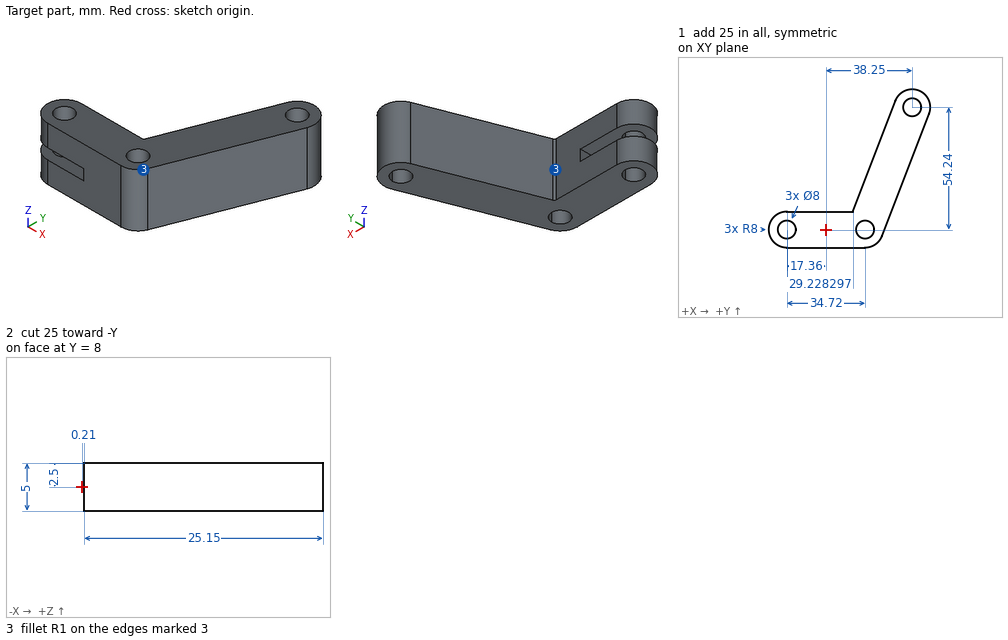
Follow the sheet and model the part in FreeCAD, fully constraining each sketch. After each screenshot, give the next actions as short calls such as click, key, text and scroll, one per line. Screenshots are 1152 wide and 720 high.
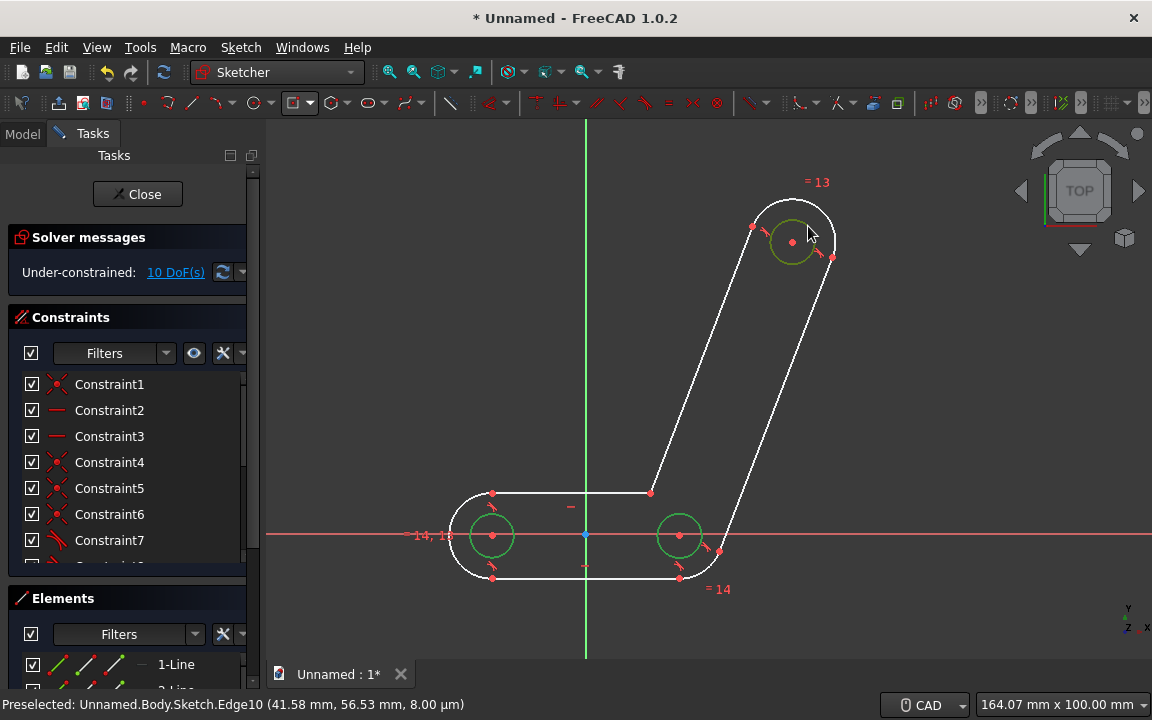
click(670, 104)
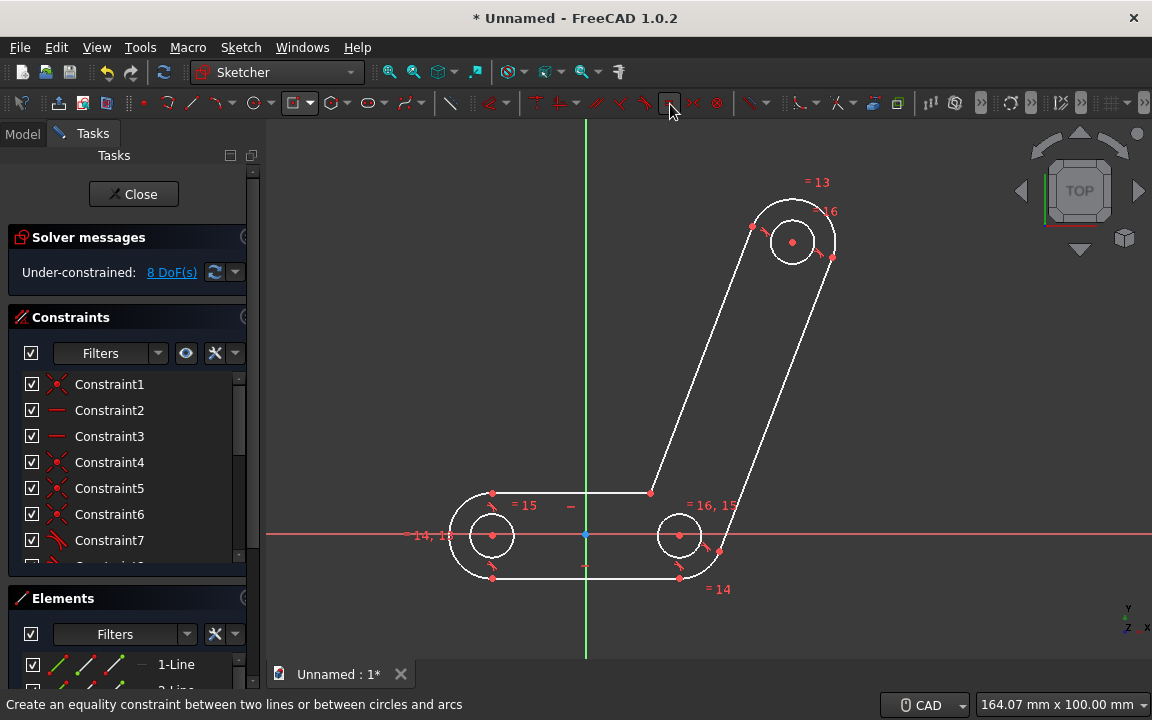
click(492, 536)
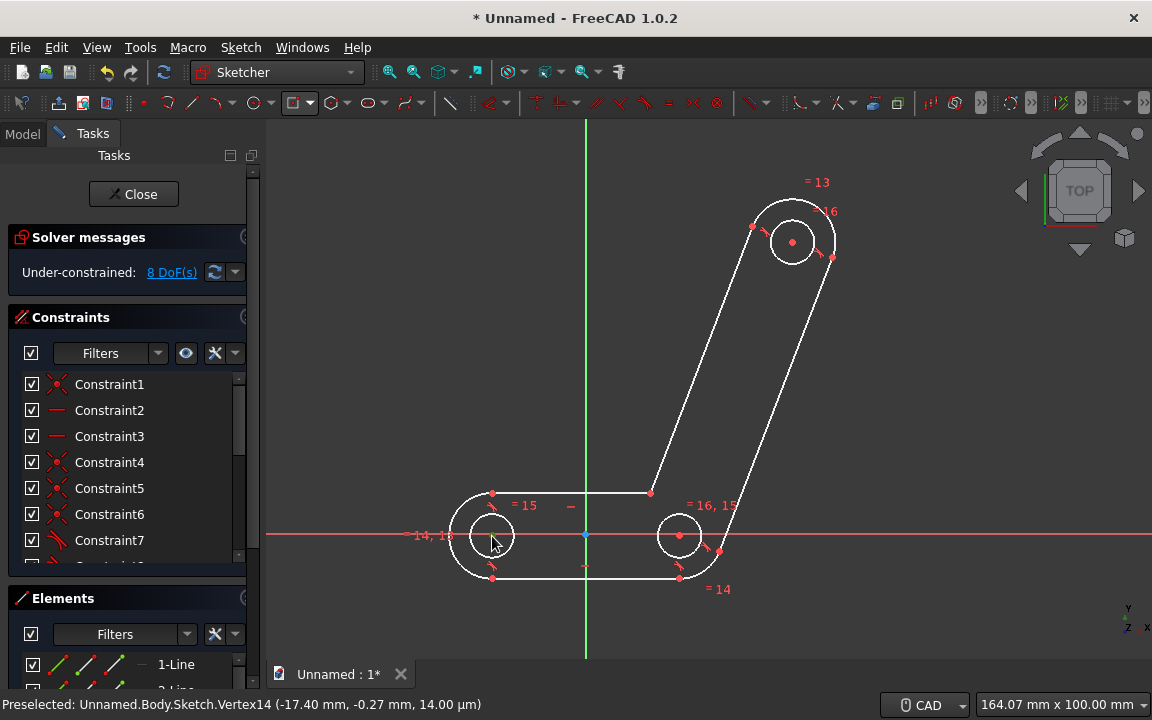
click(344, 534)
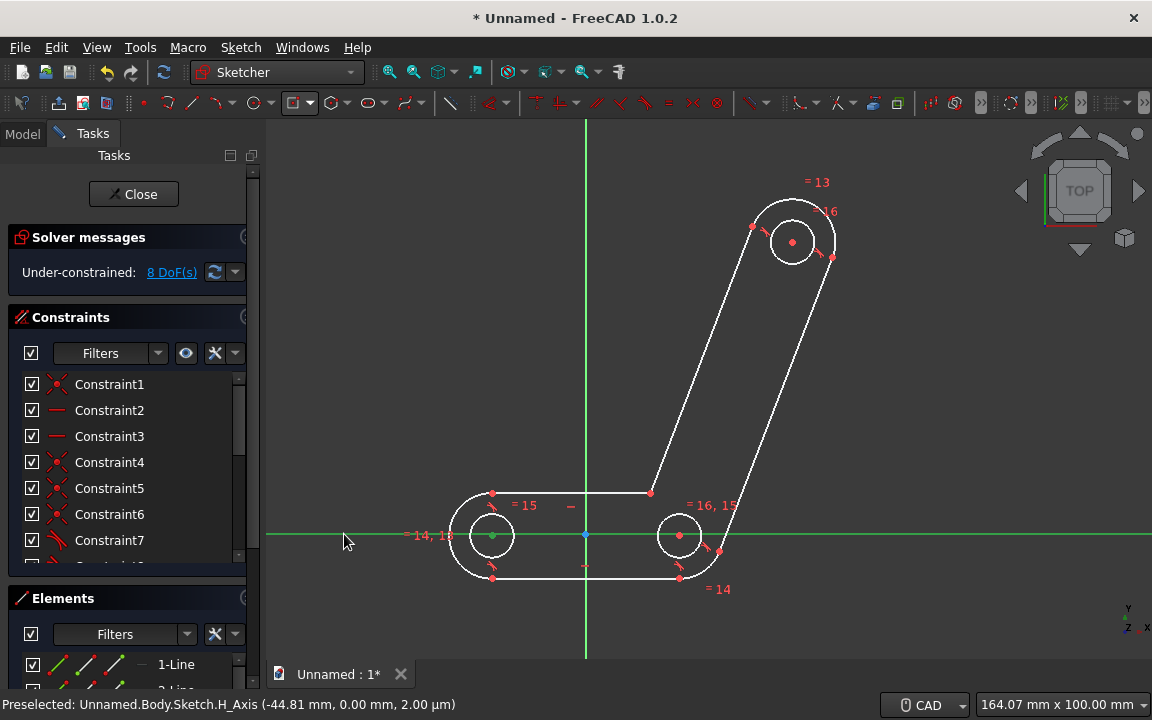
click(536, 104)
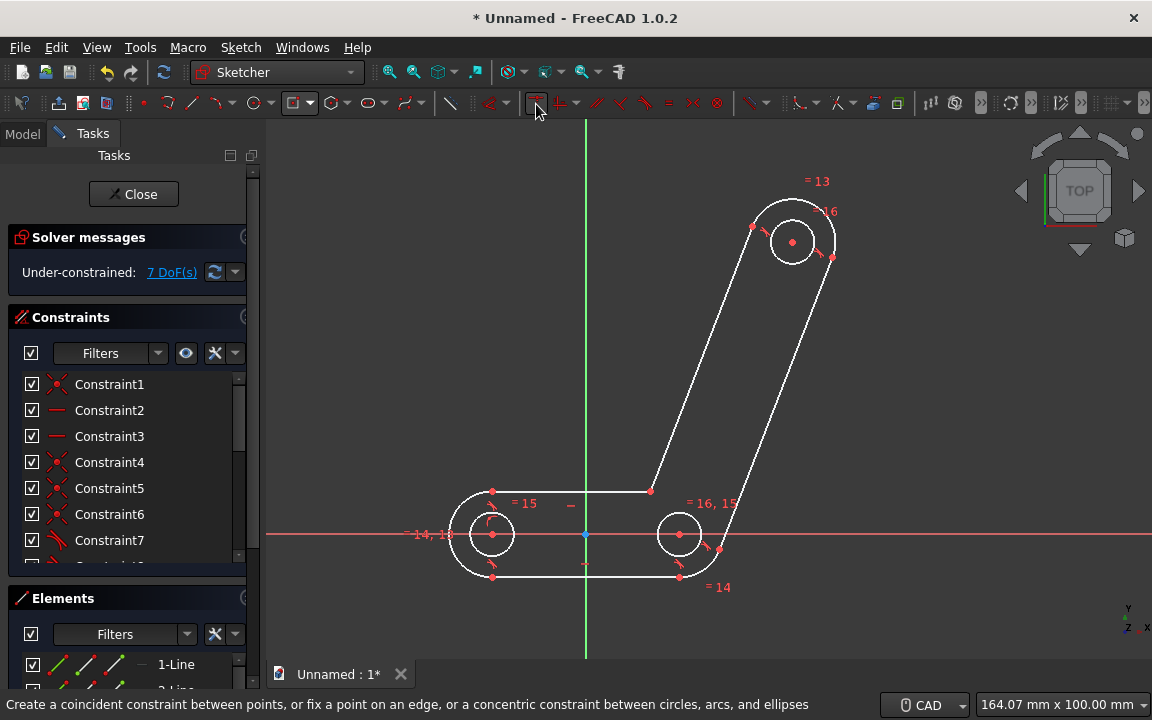
click(829, 219)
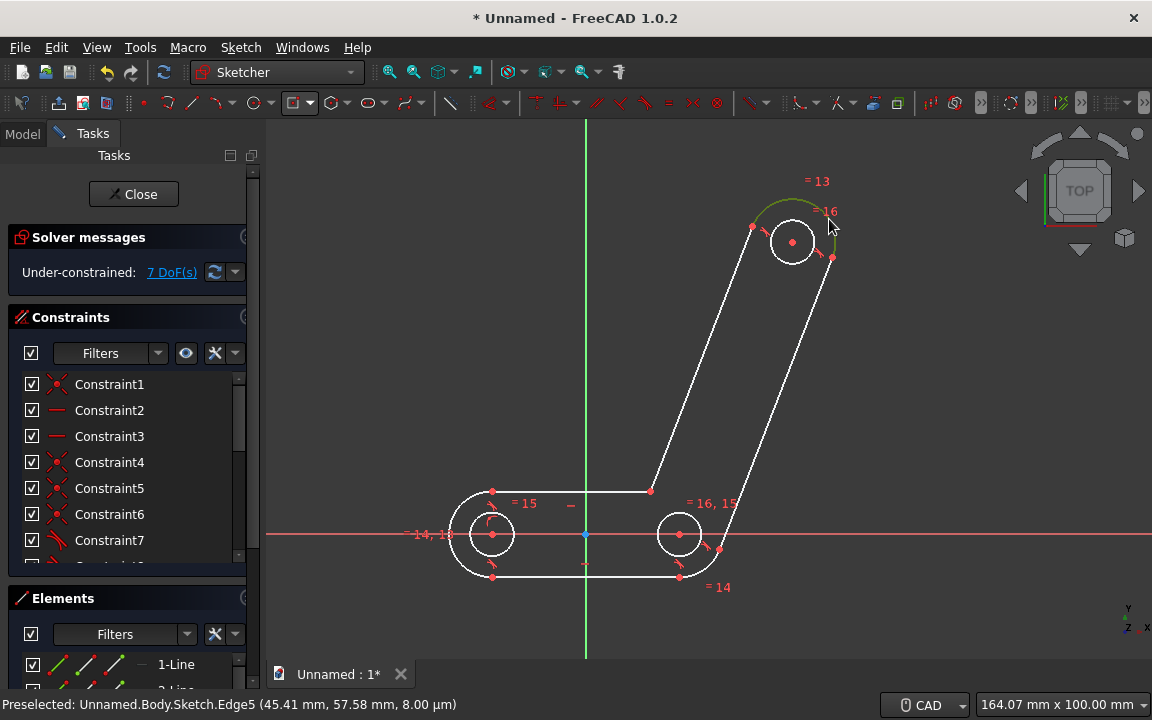
click(508, 104)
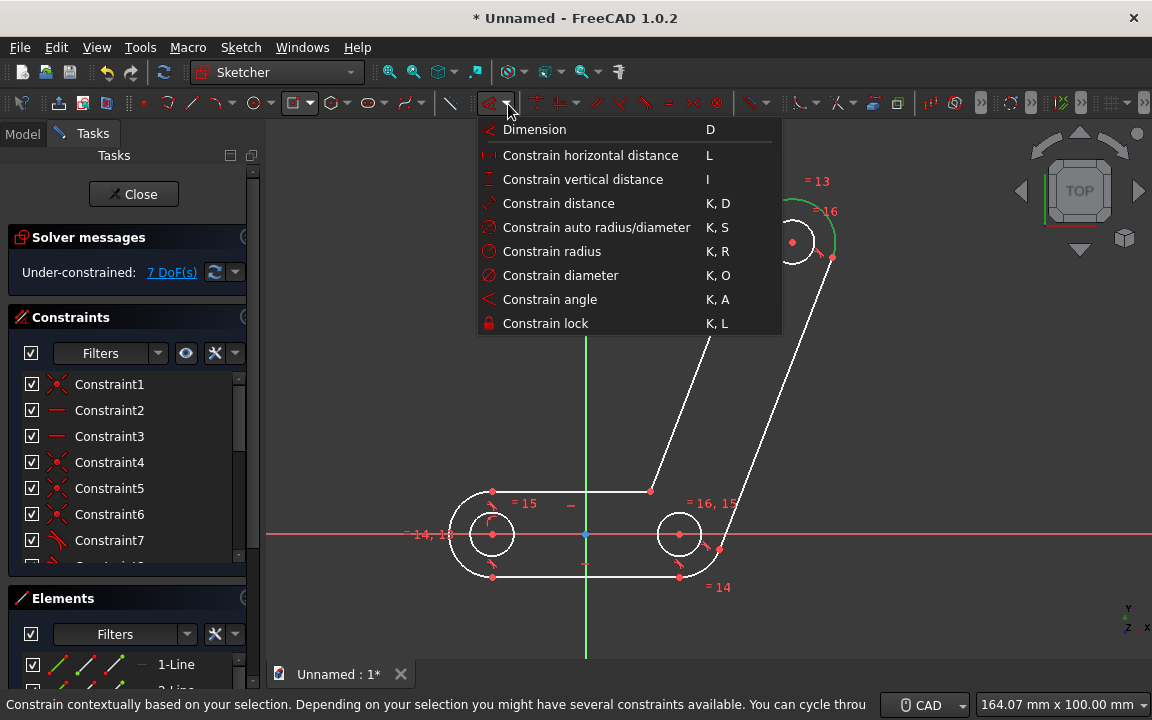
click(630, 251)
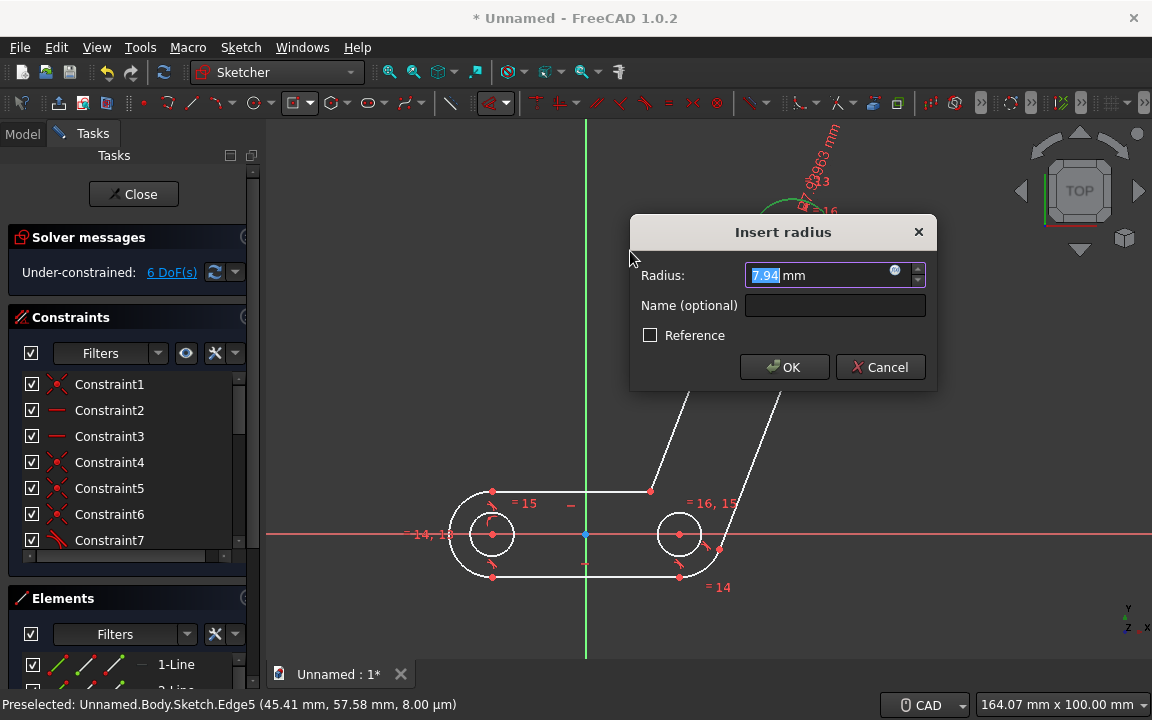
text(8)
key(Return)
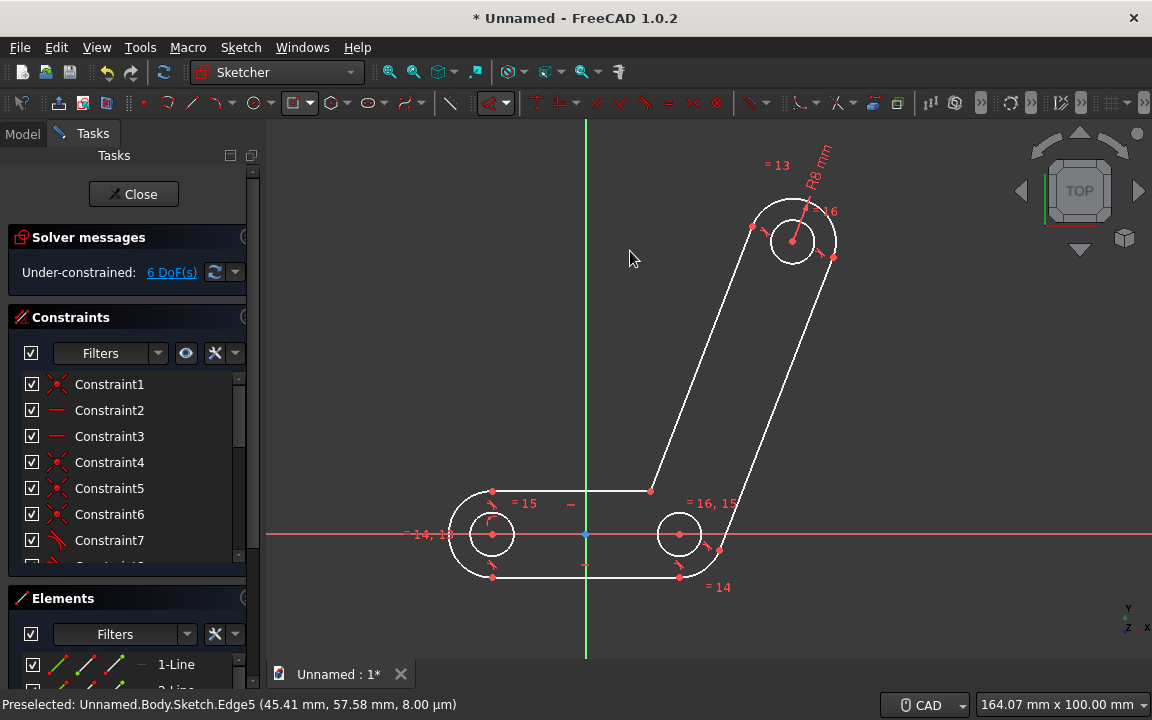
click(507, 519)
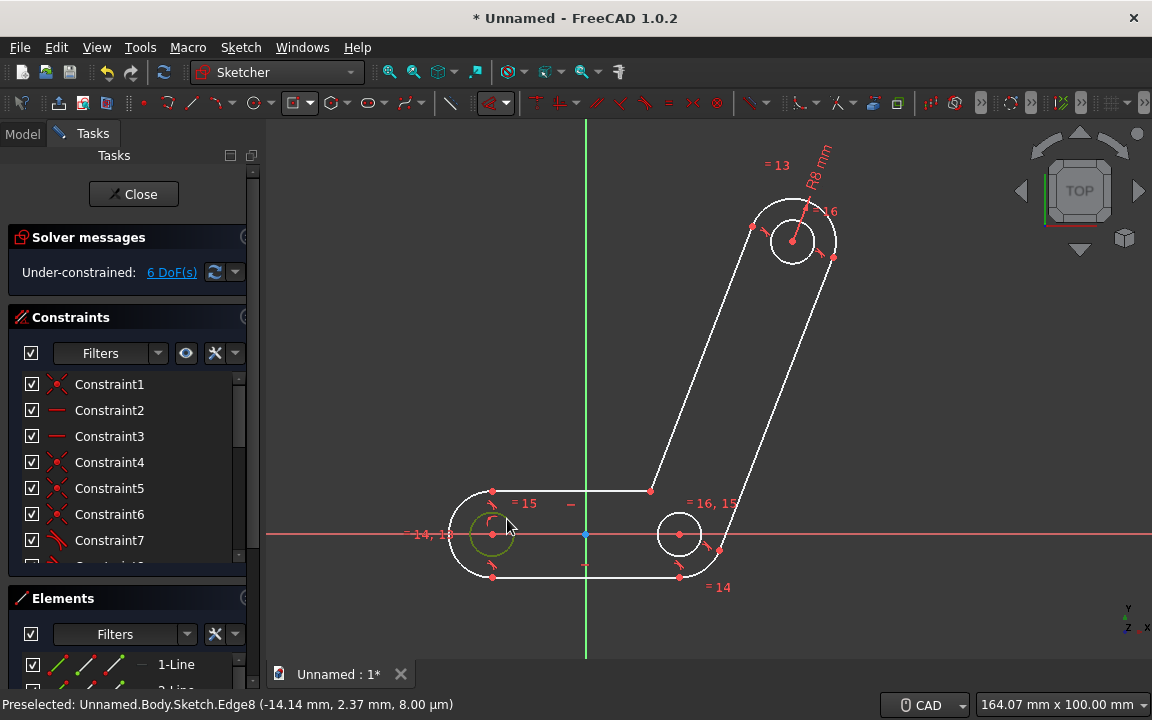
key(k)
key(o)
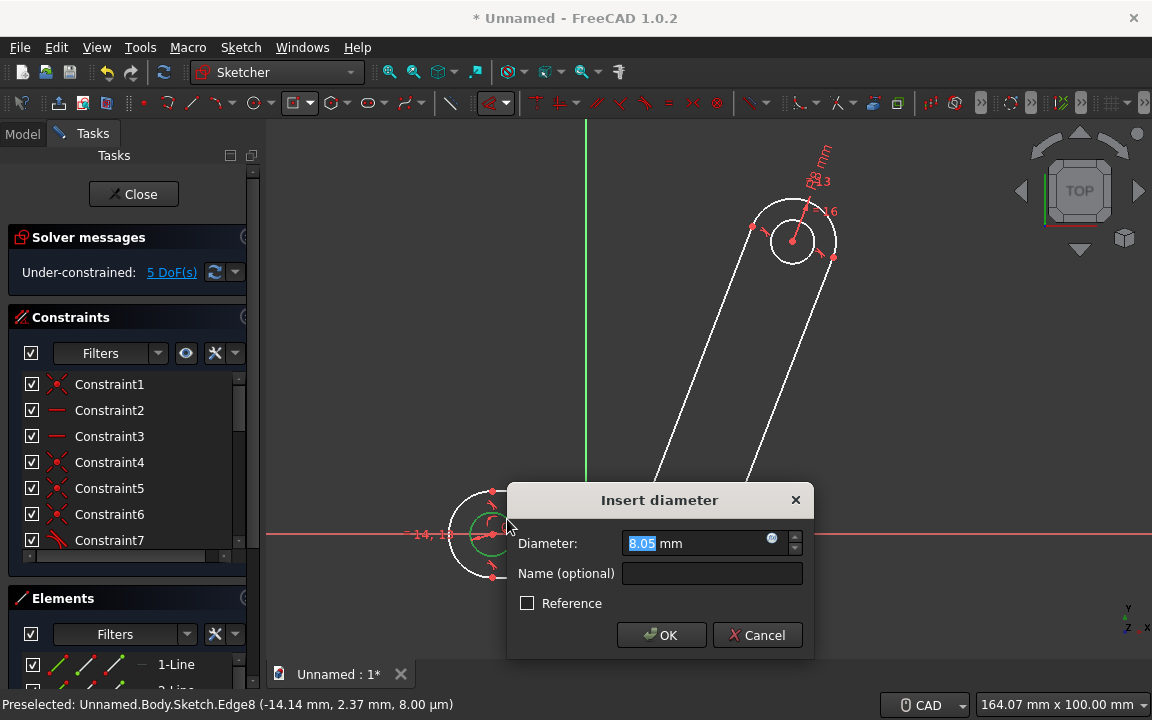
text(8)
key(Return)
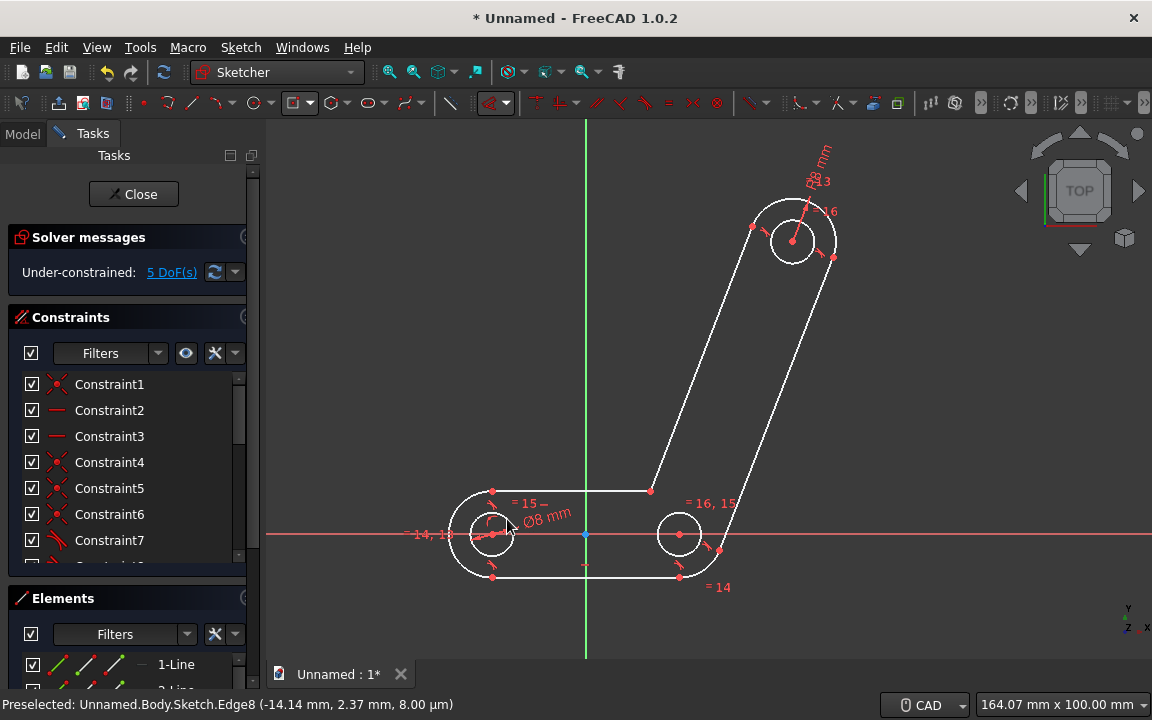
click(548, 578)